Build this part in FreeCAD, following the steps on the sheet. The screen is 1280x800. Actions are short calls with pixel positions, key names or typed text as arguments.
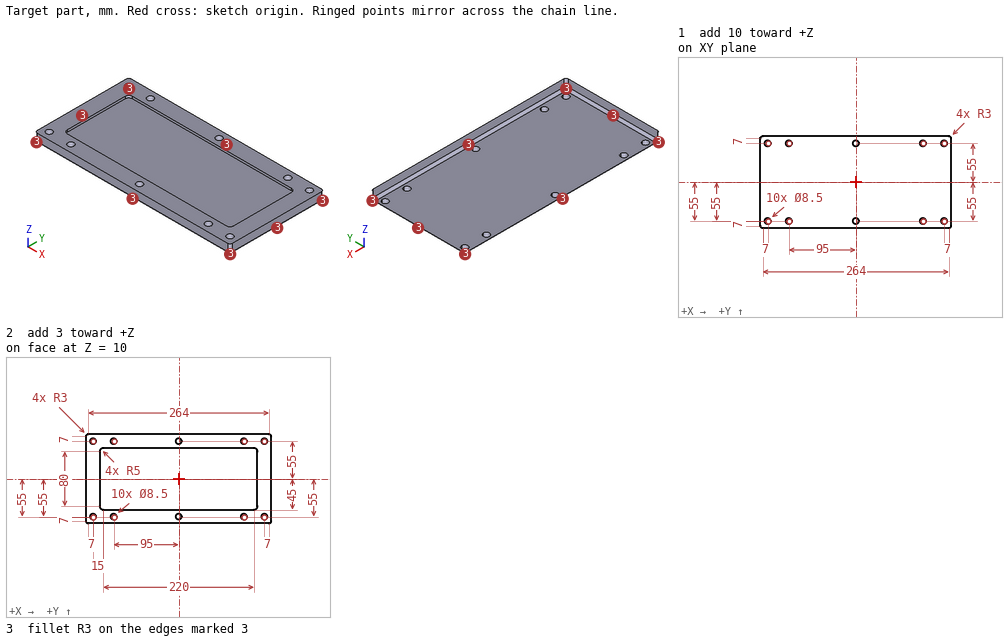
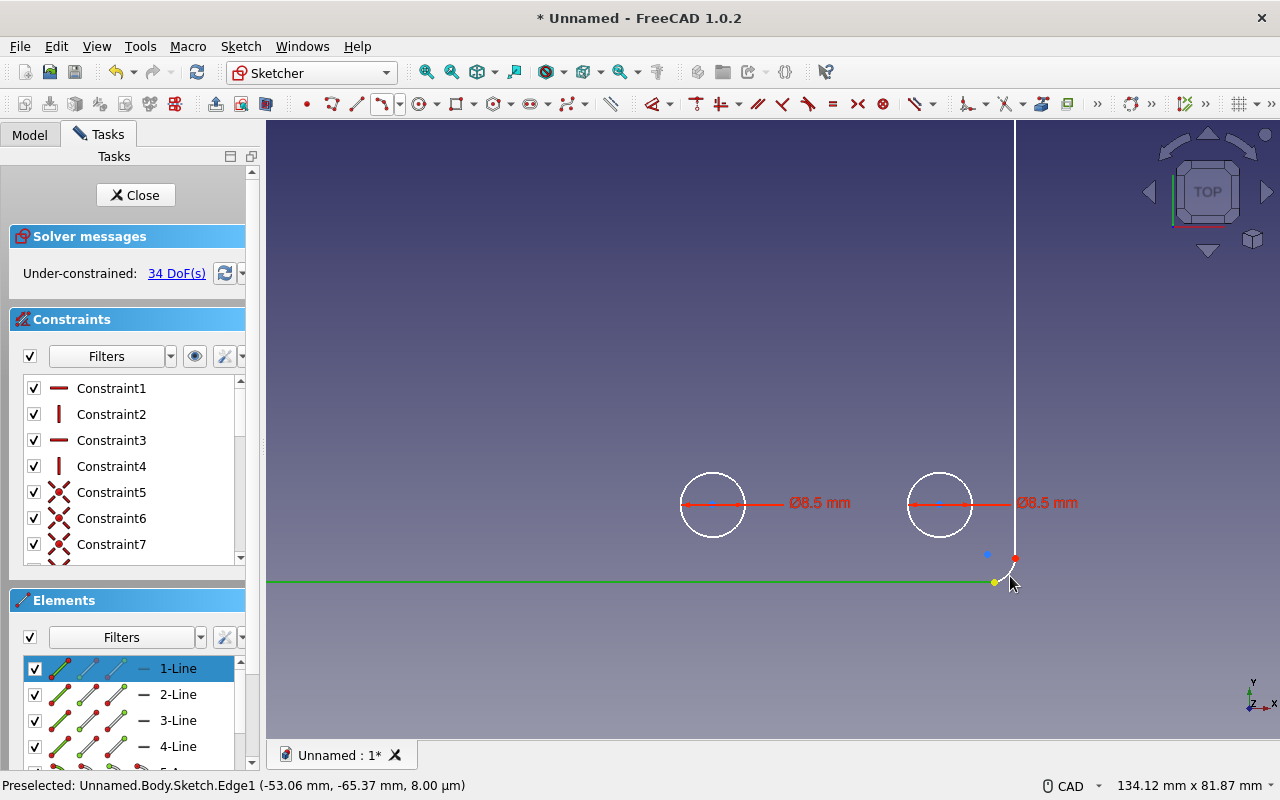
click(1009, 574)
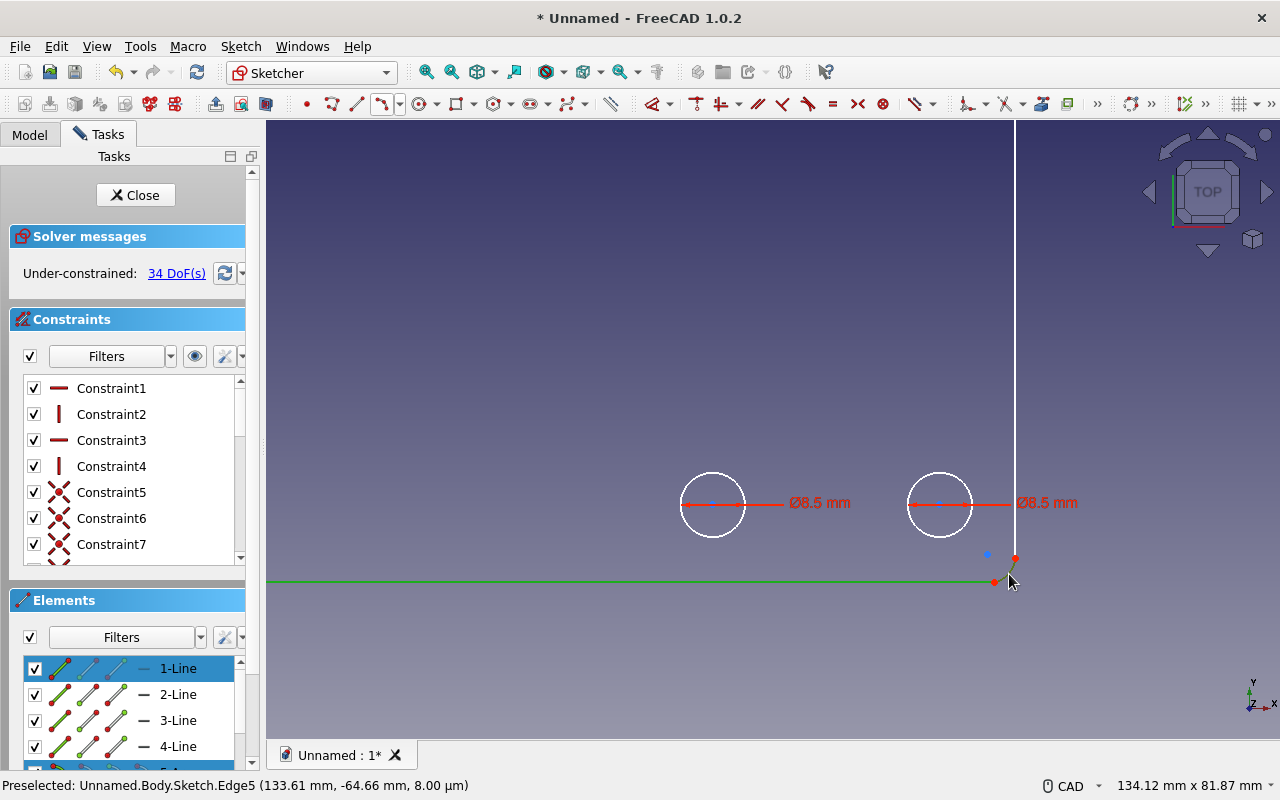
click(808, 104)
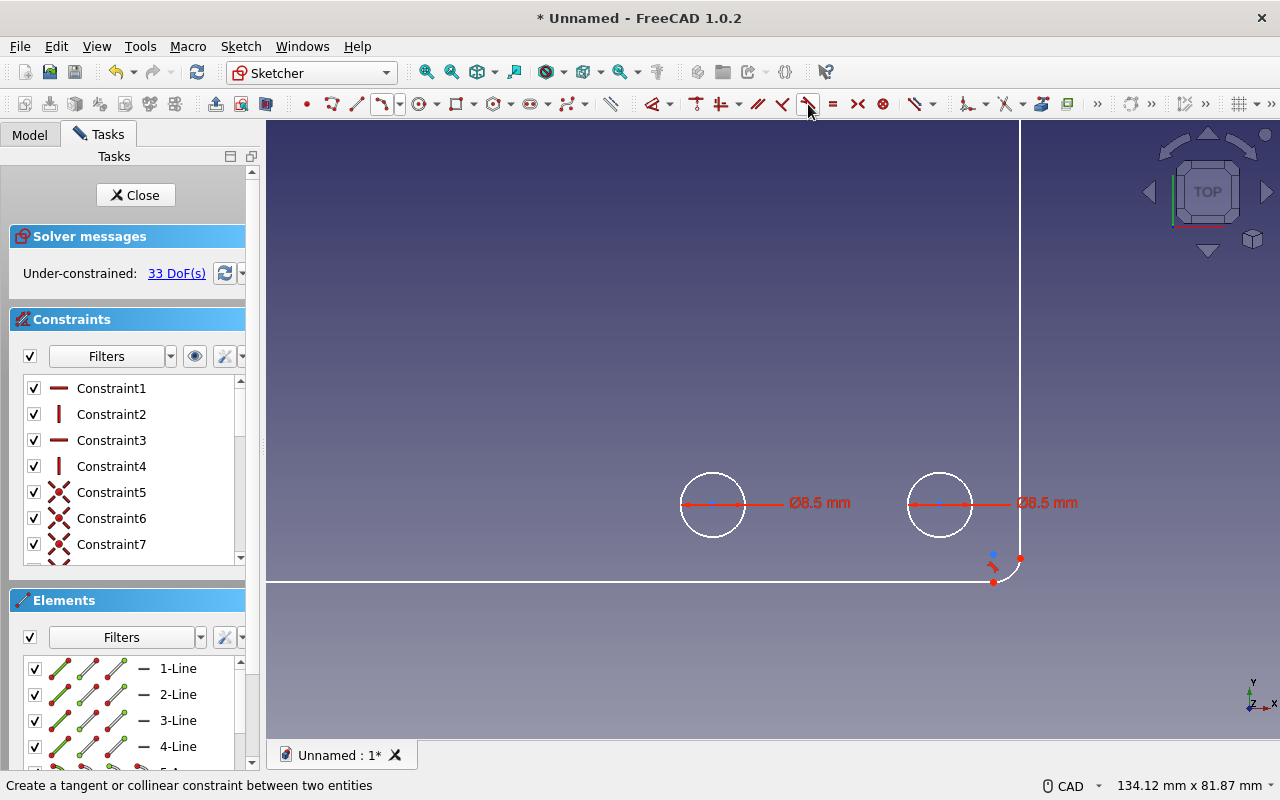
click(394, 582)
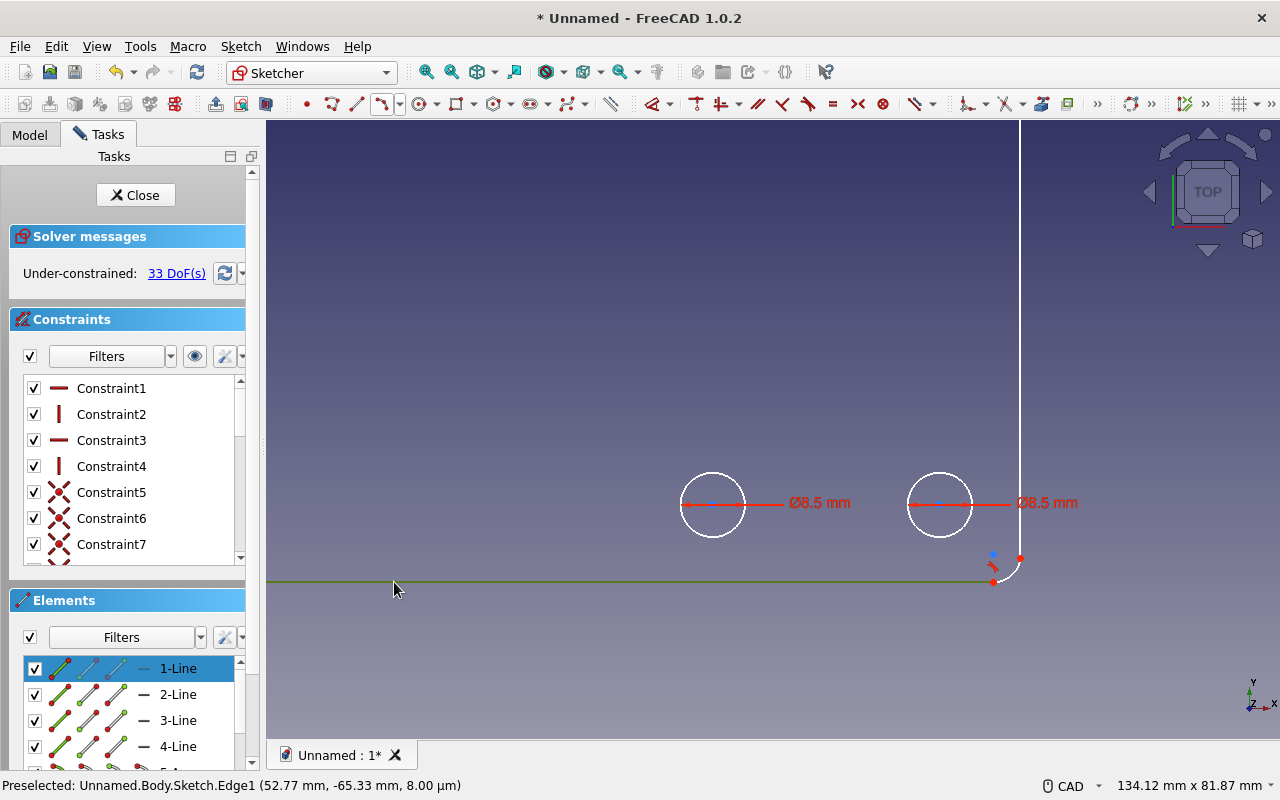
scroll(1010, 577, down, 6)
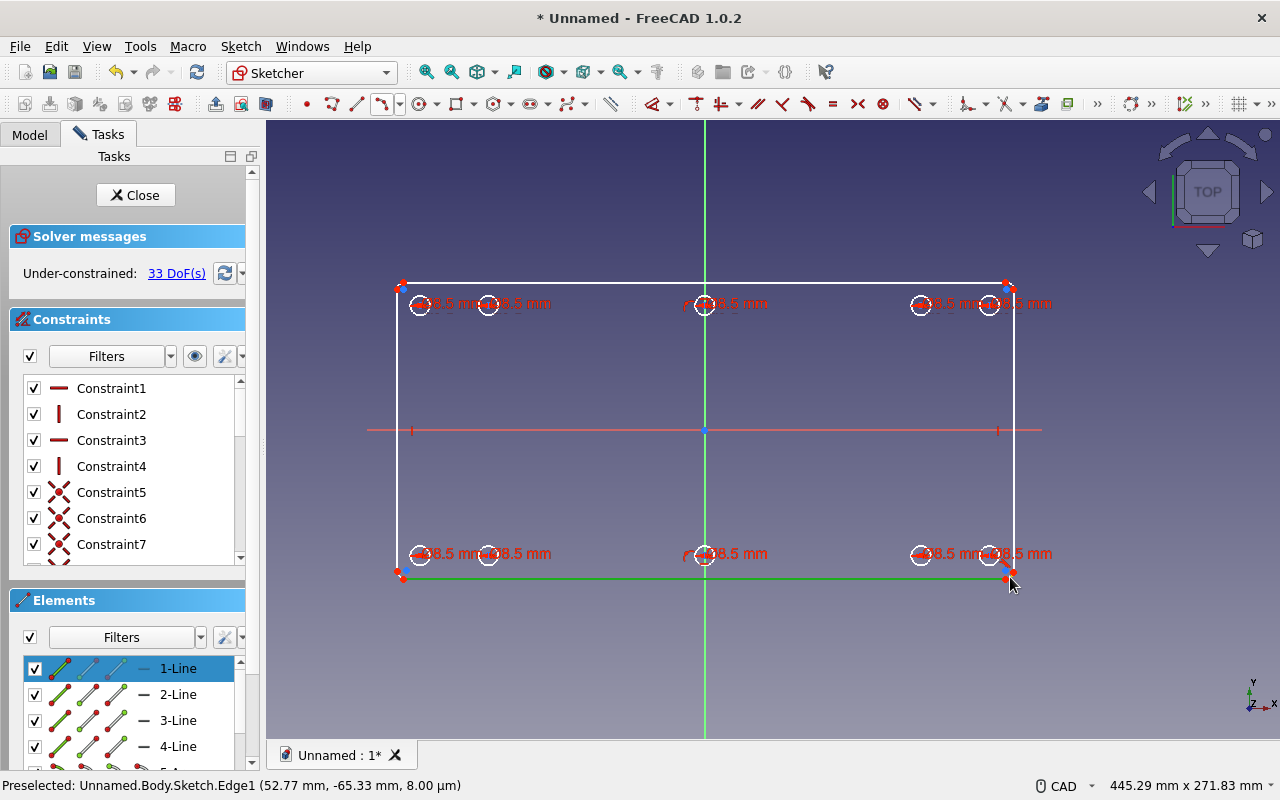
scroll(398, 575, up, 8)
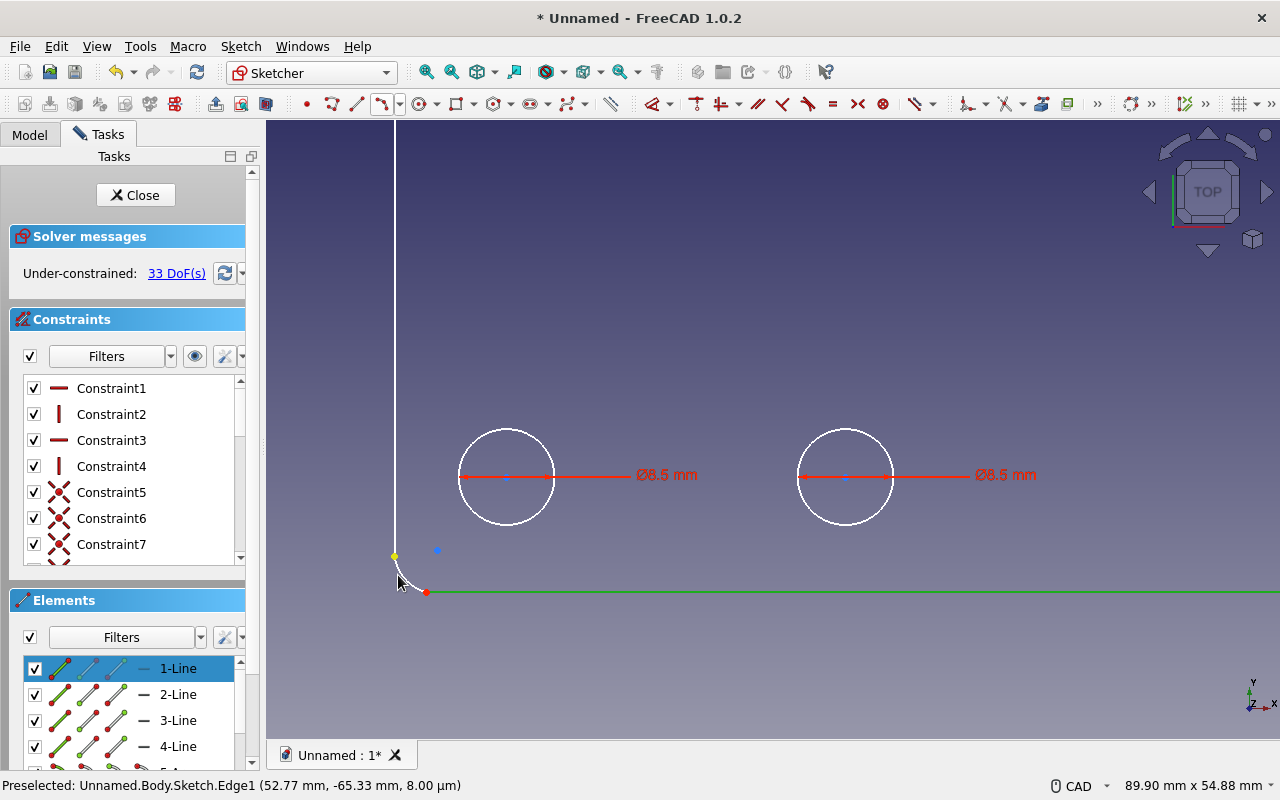
click(400, 571)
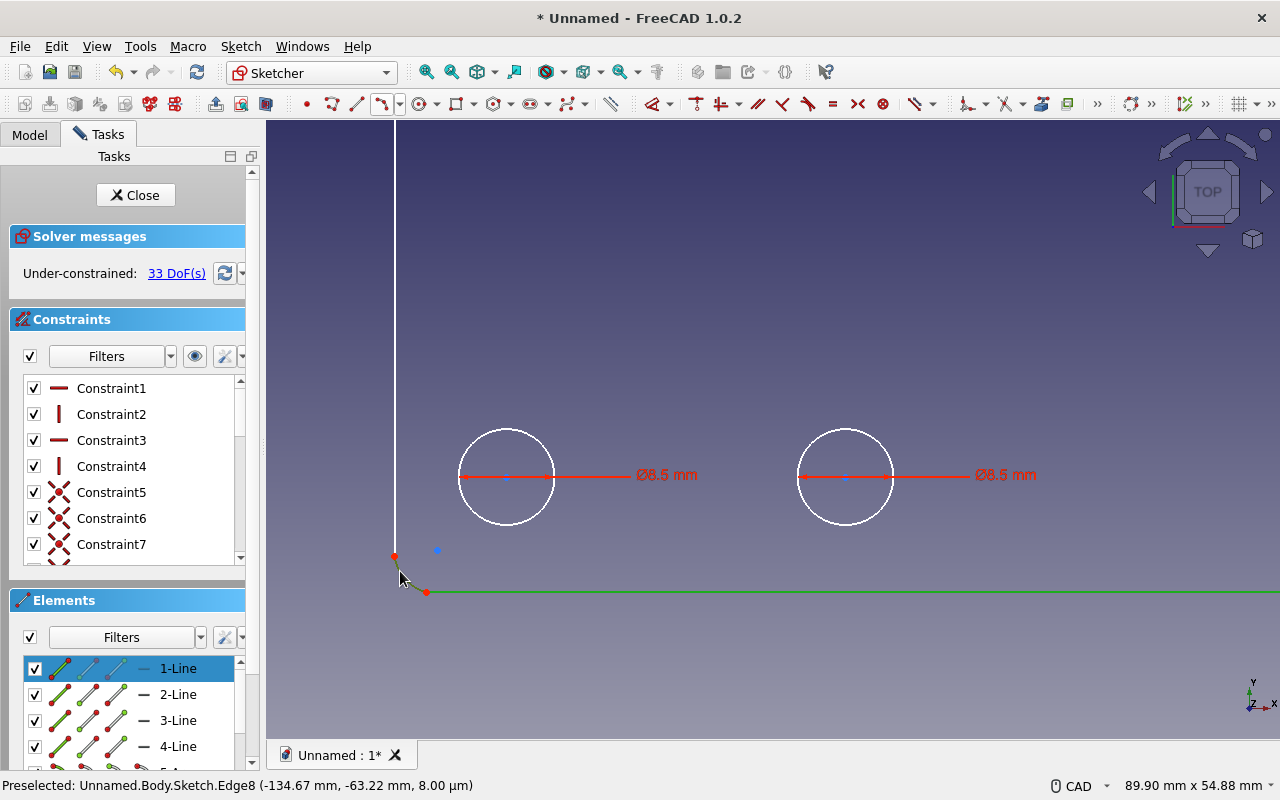
click(808, 104)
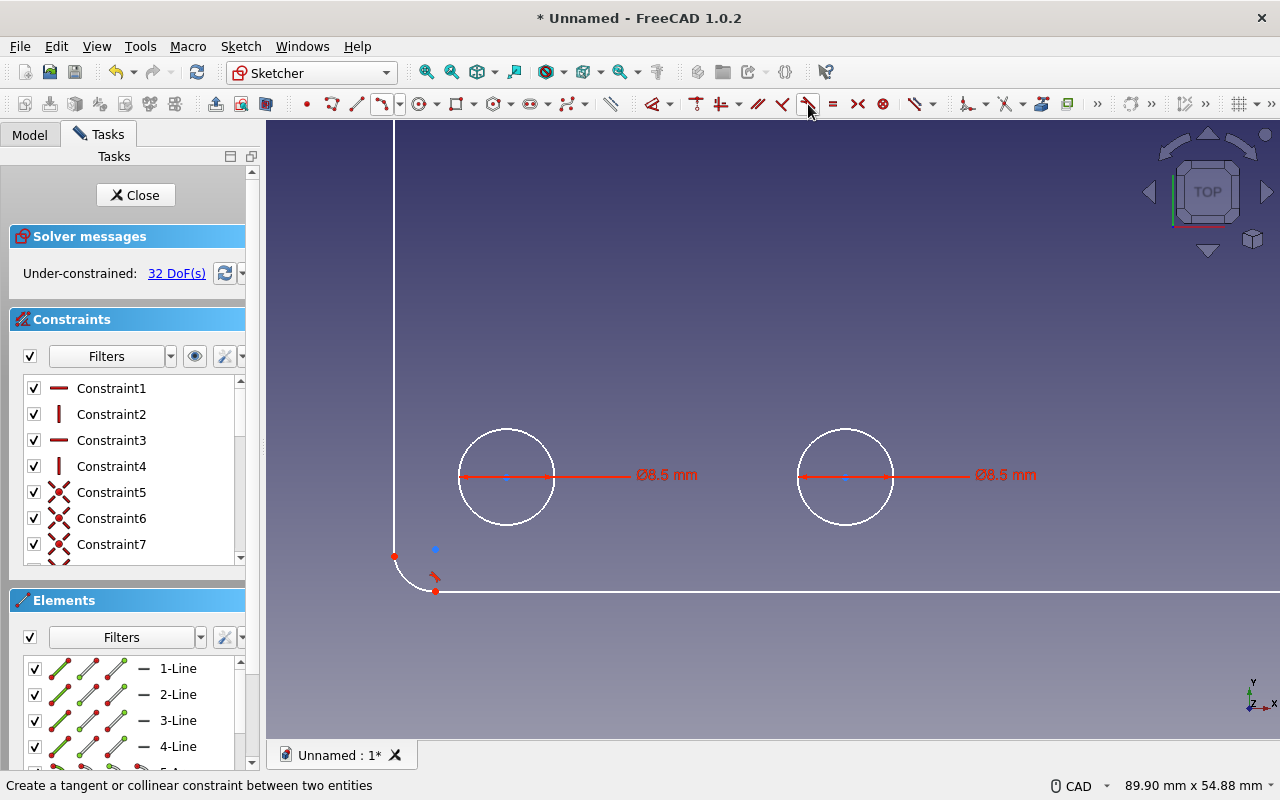
scroll(398, 575, down, 8)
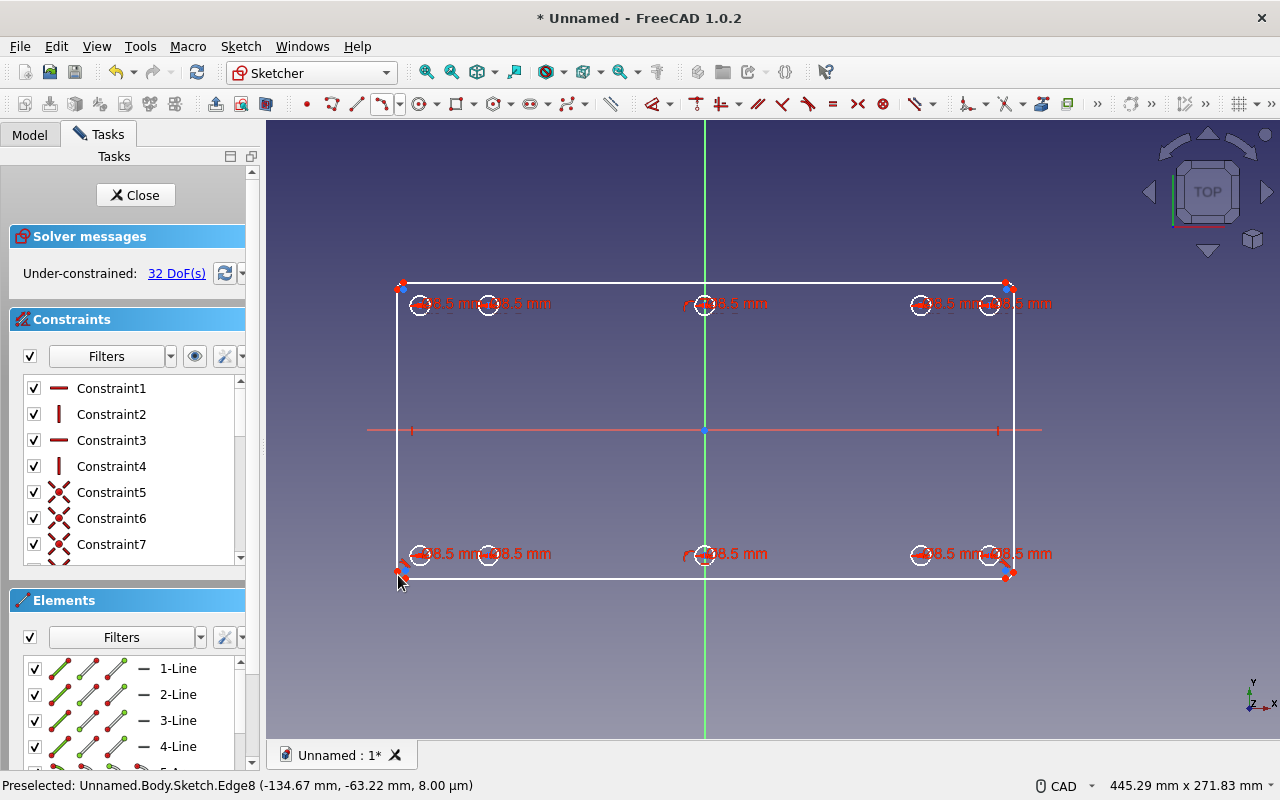
click(1014, 487)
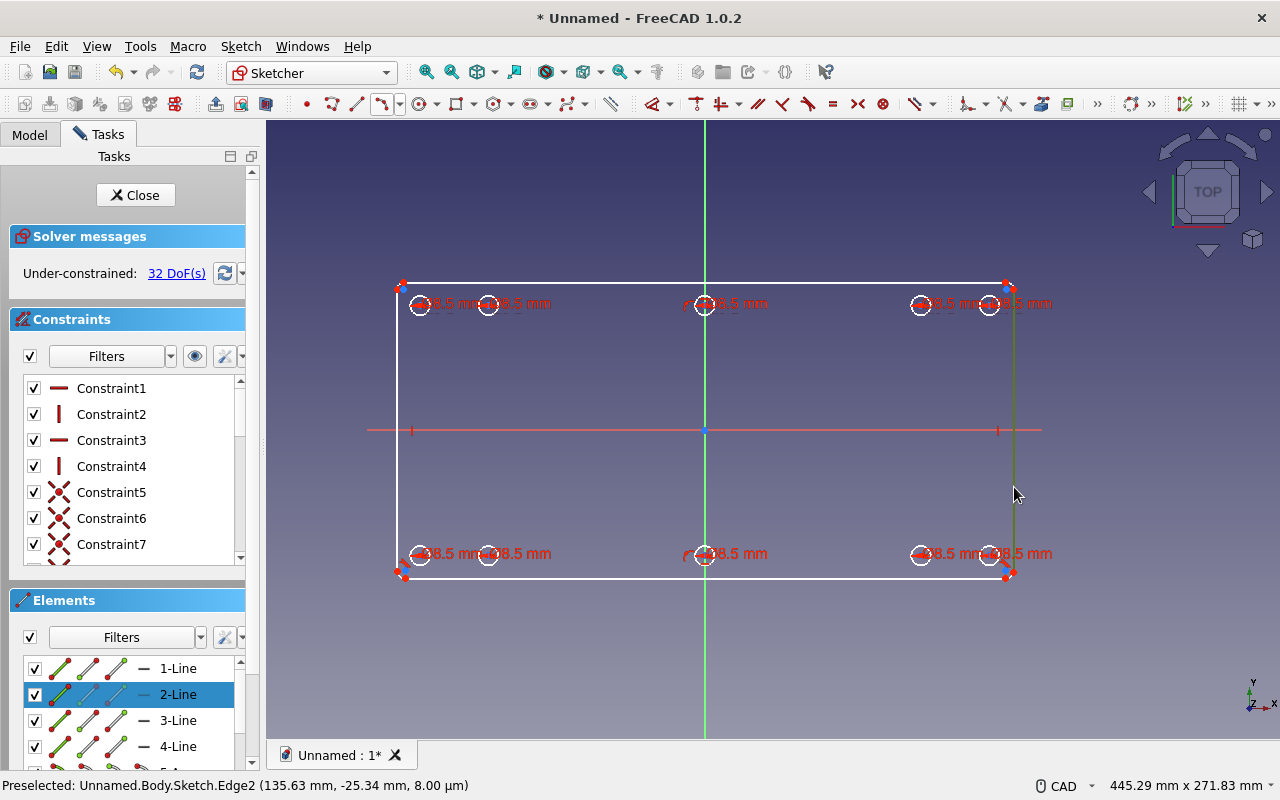
scroll(1011, 577, up, 5)